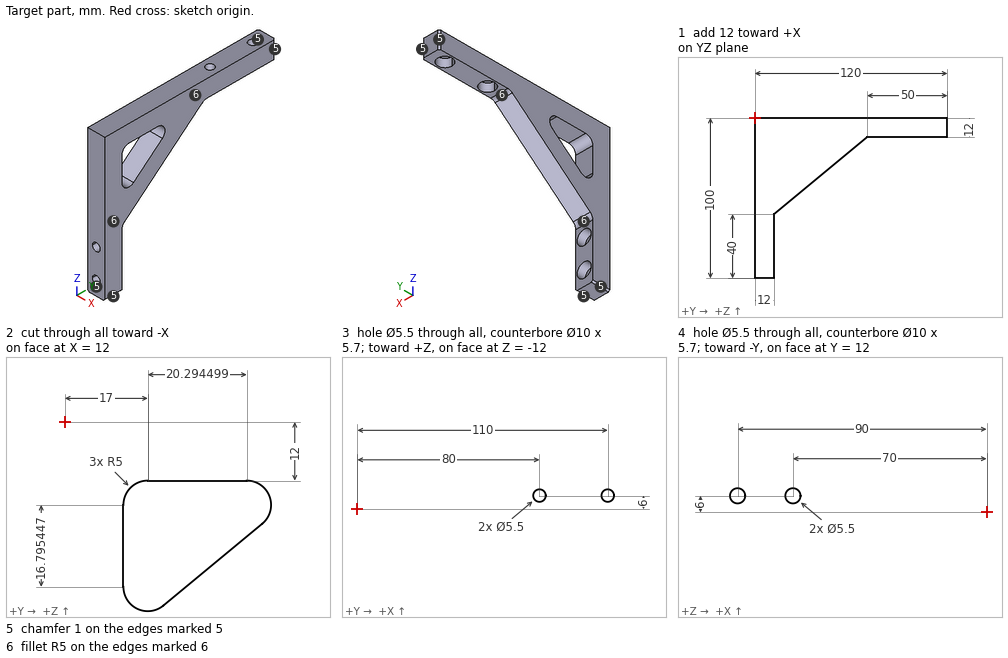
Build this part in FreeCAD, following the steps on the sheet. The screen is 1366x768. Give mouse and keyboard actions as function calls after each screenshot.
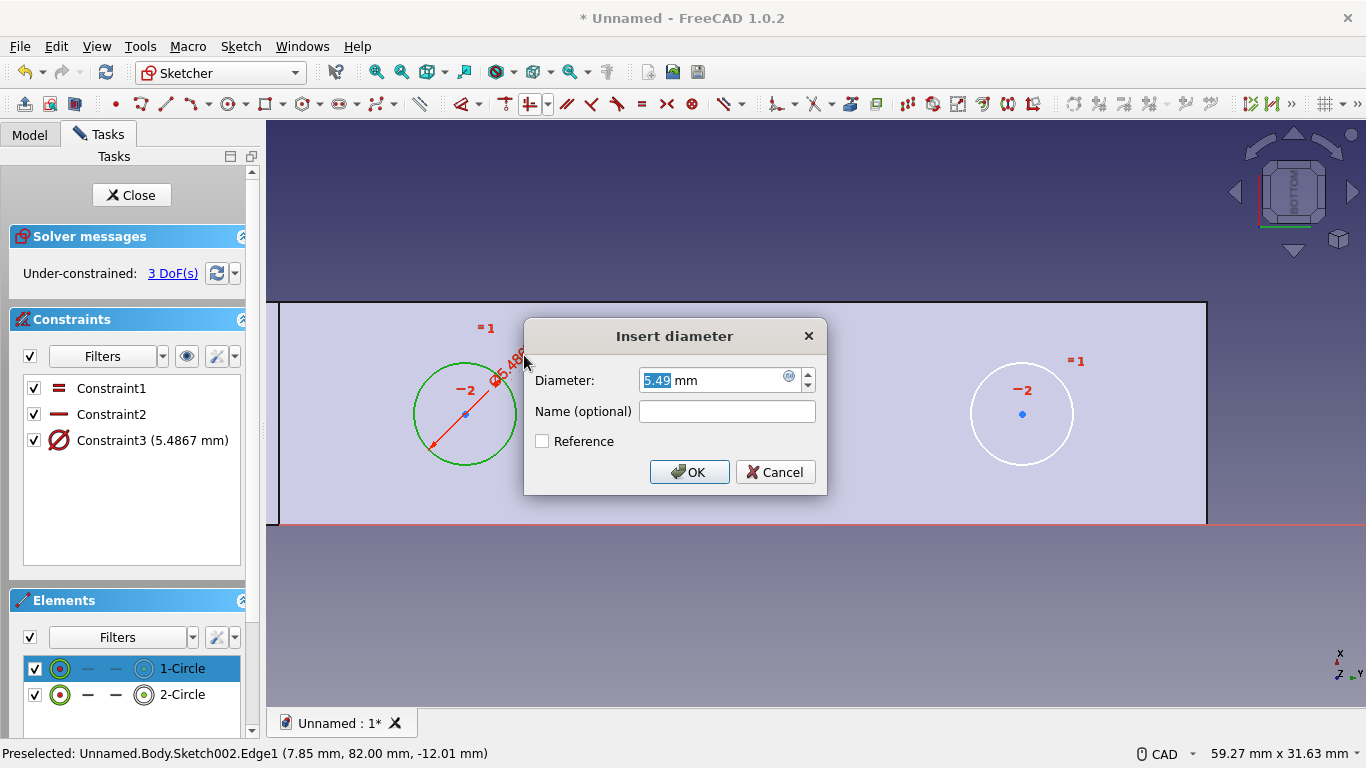
text(5.5)
key(Return)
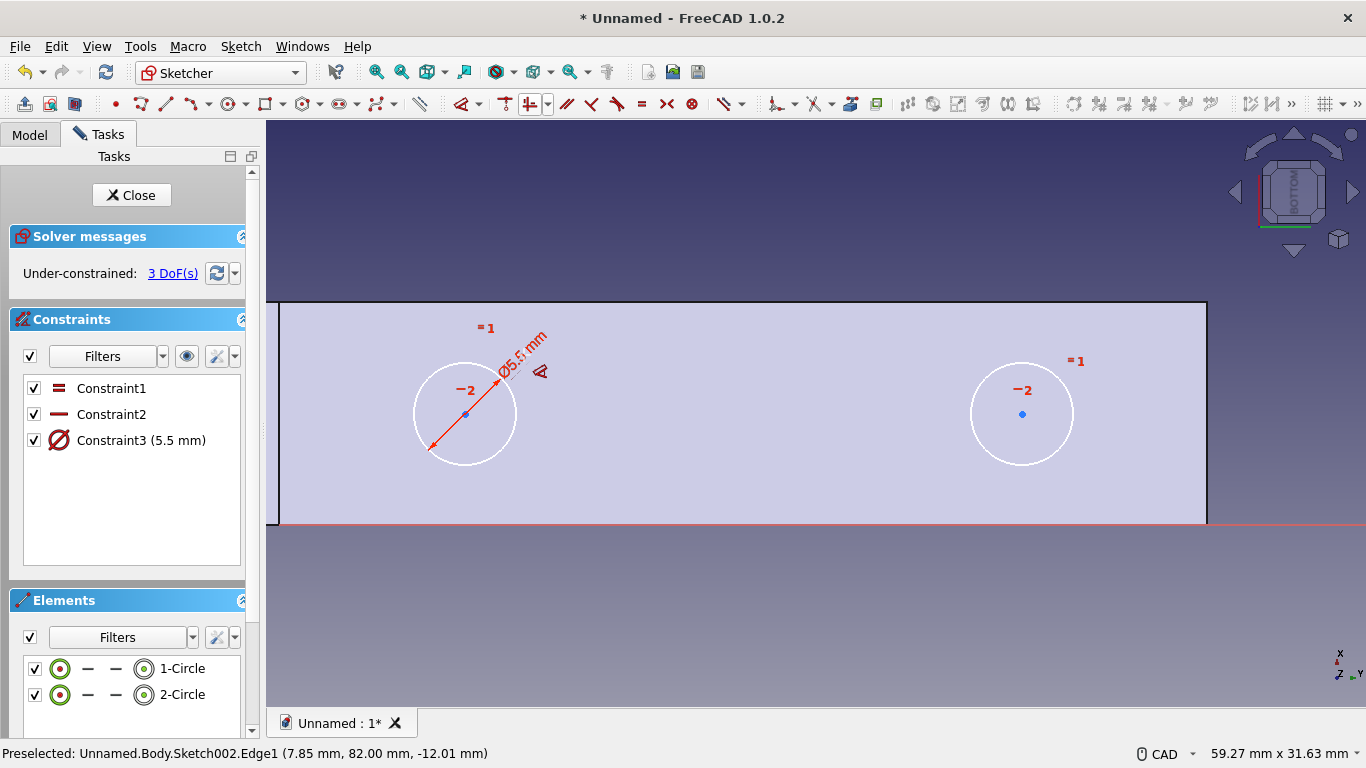
click(465, 414)
click(499, 469)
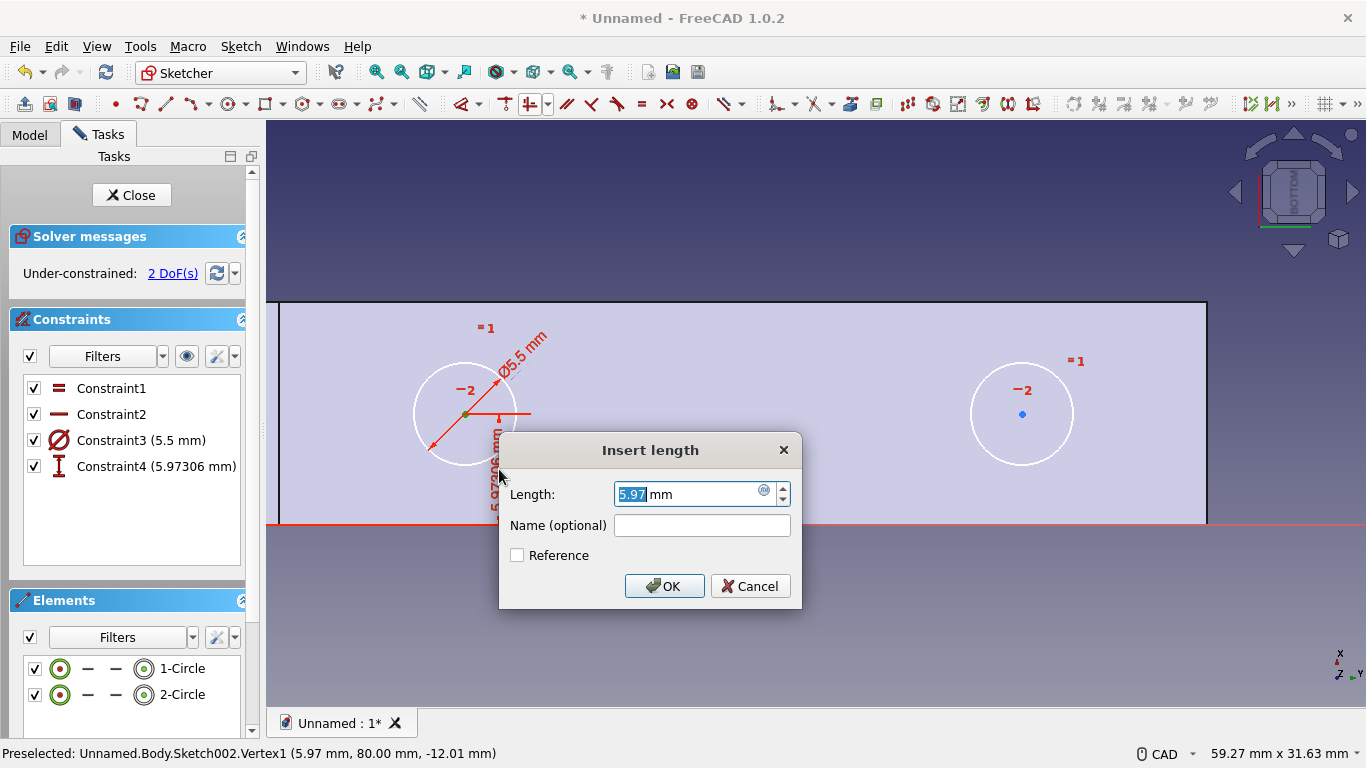
text(6)
key(Return)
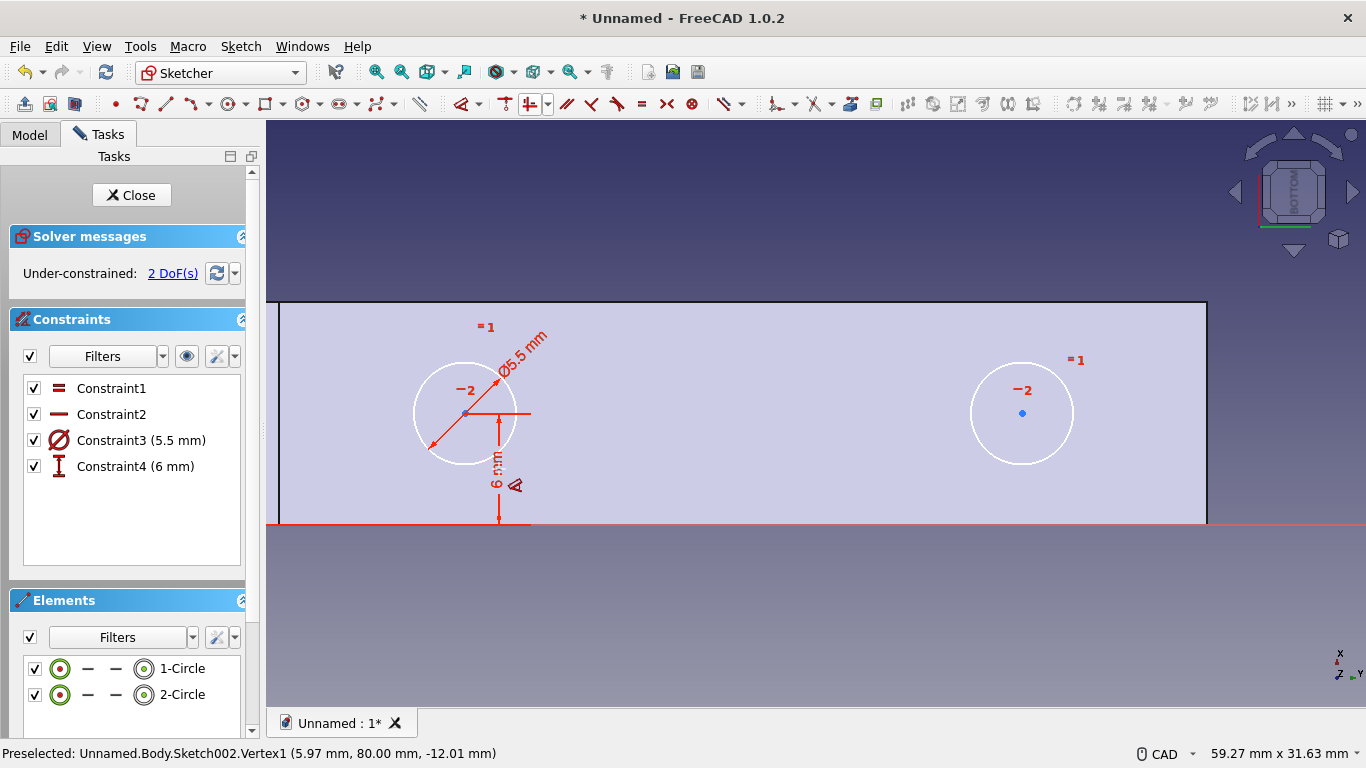
click(465, 413)
click(379, 559)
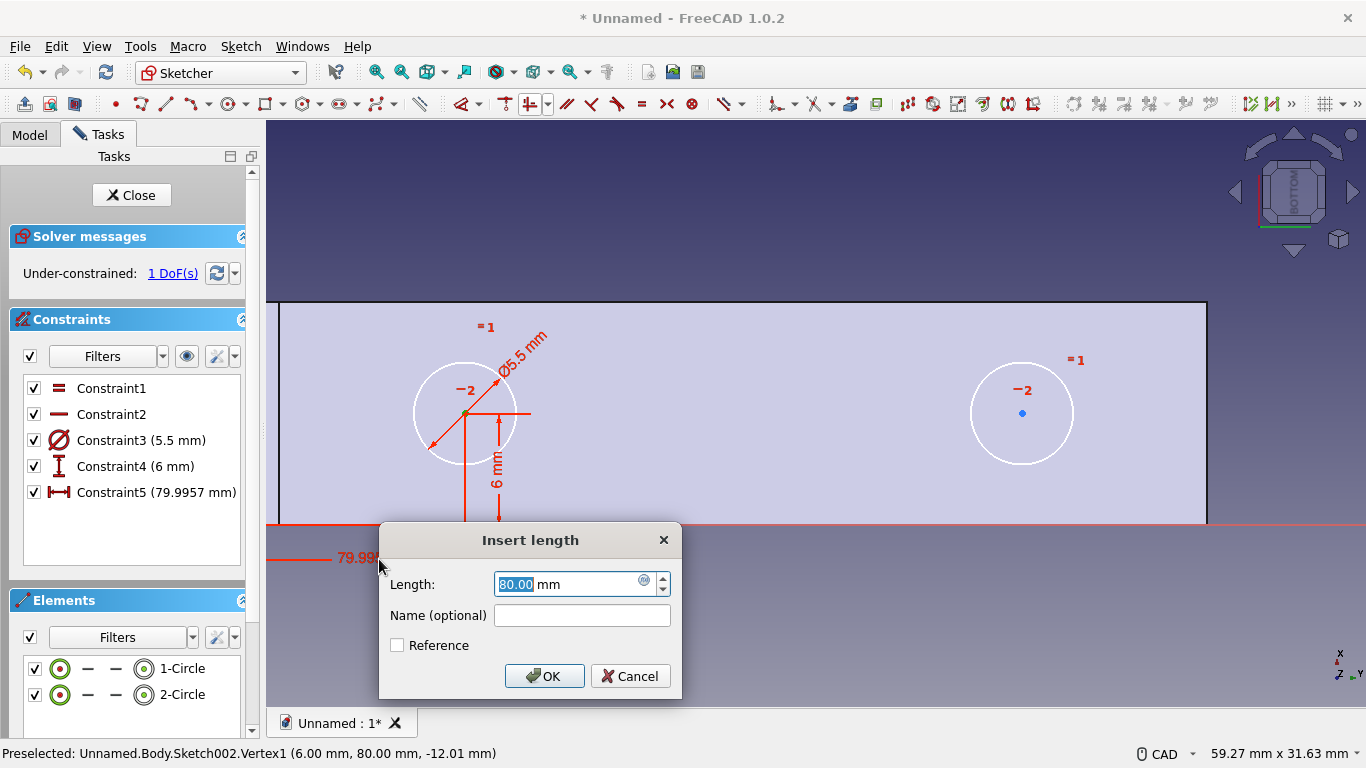
text(80)
key(Return)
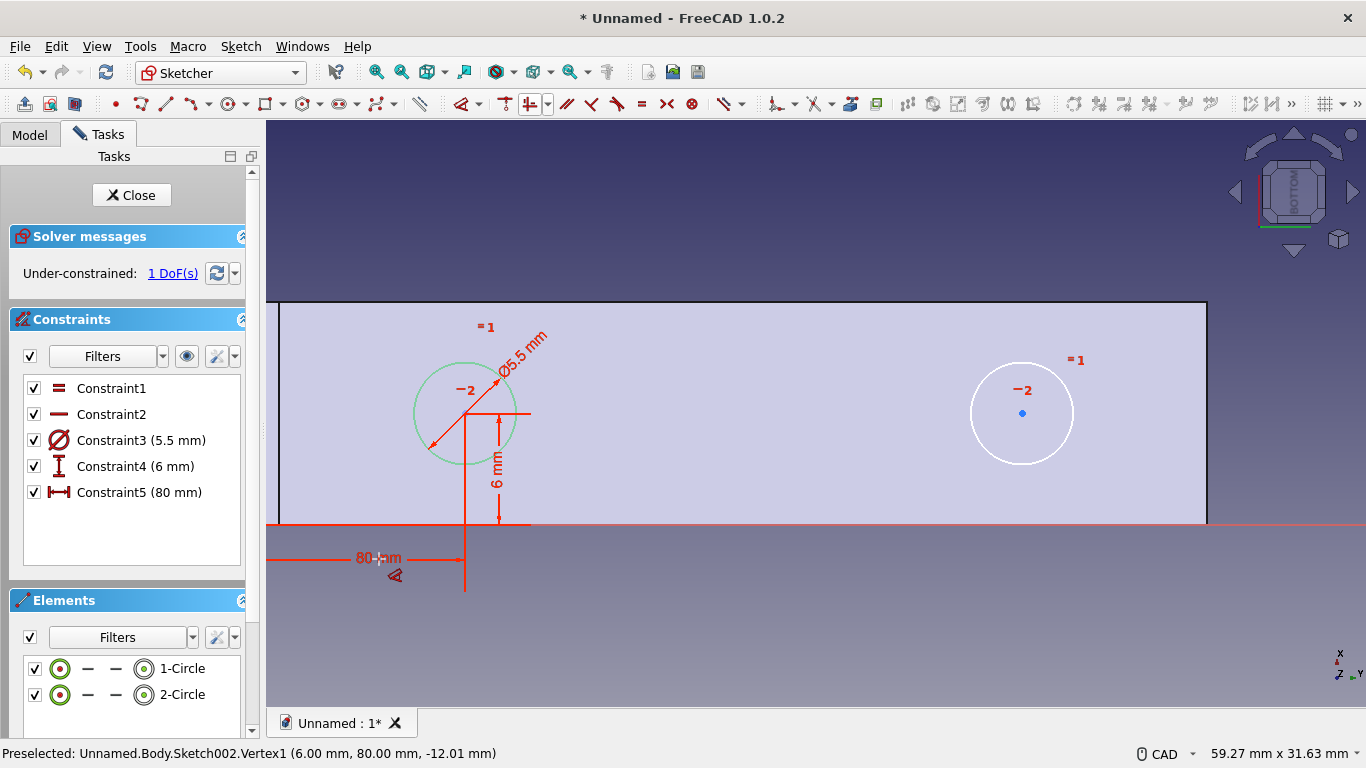
click(1022, 413)
click(658, 559)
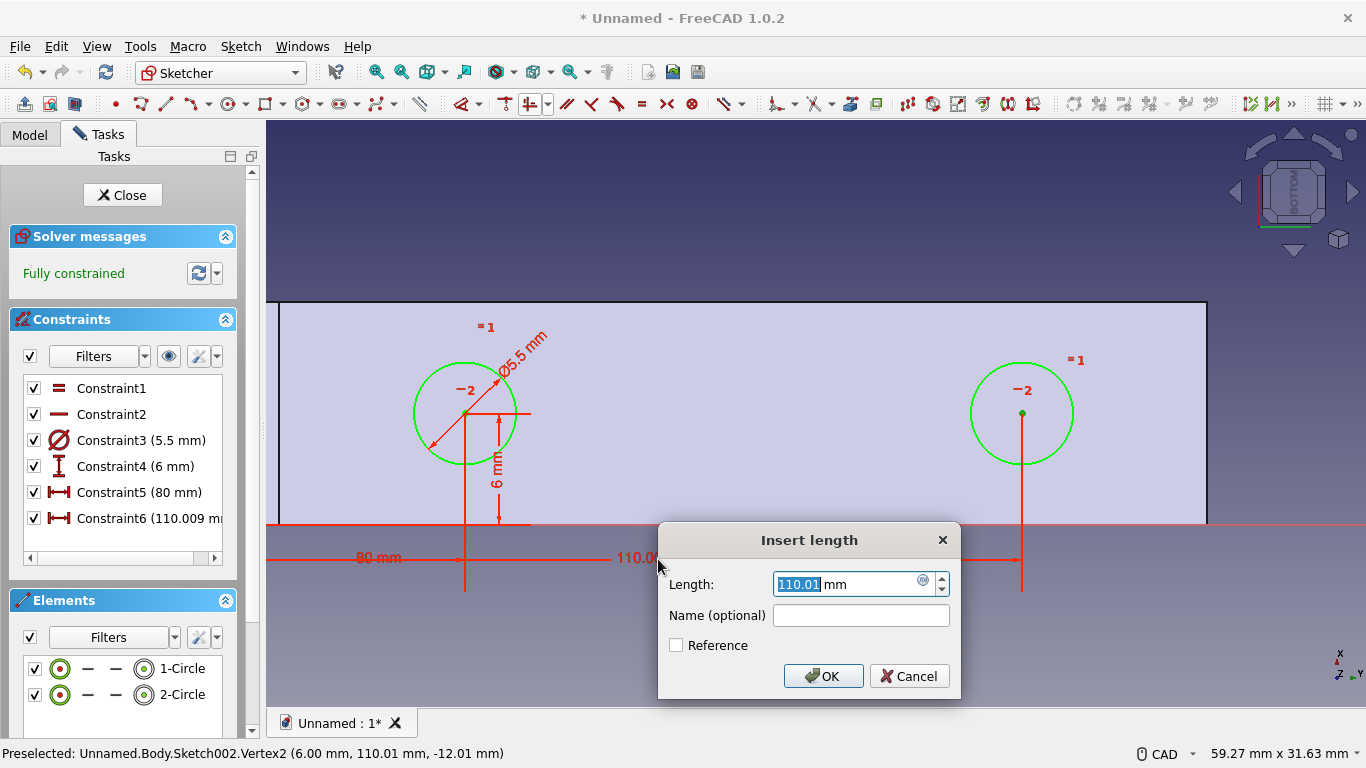
text(110)
key(Return)
key(Escape)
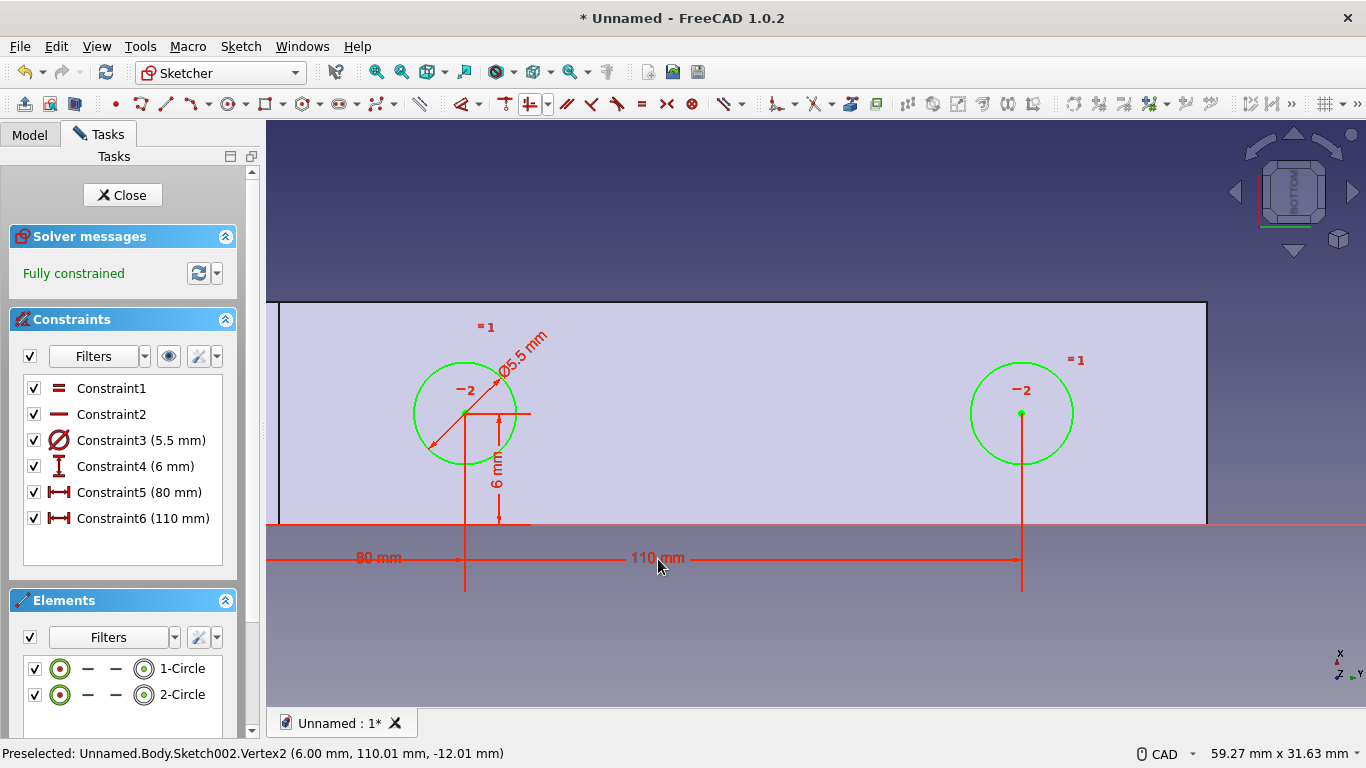
click(123, 195)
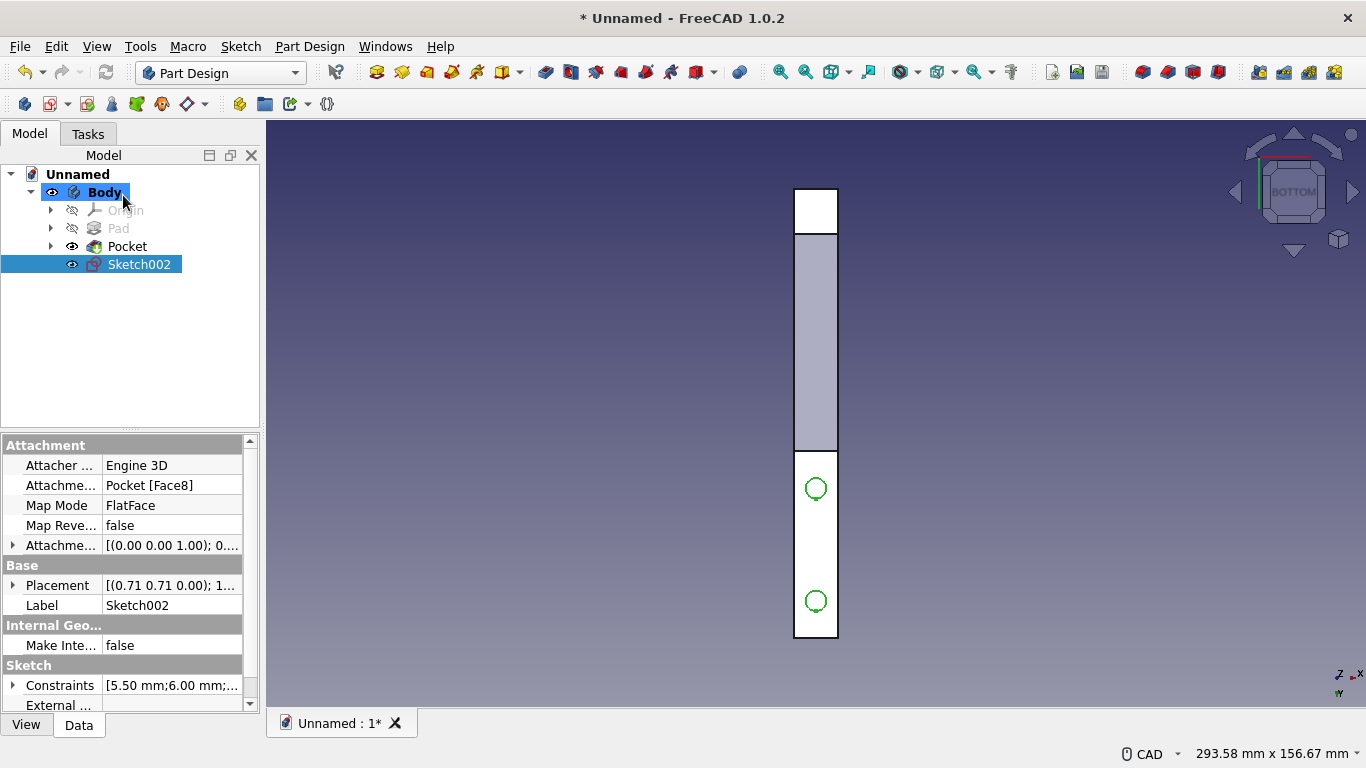
click(571, 72)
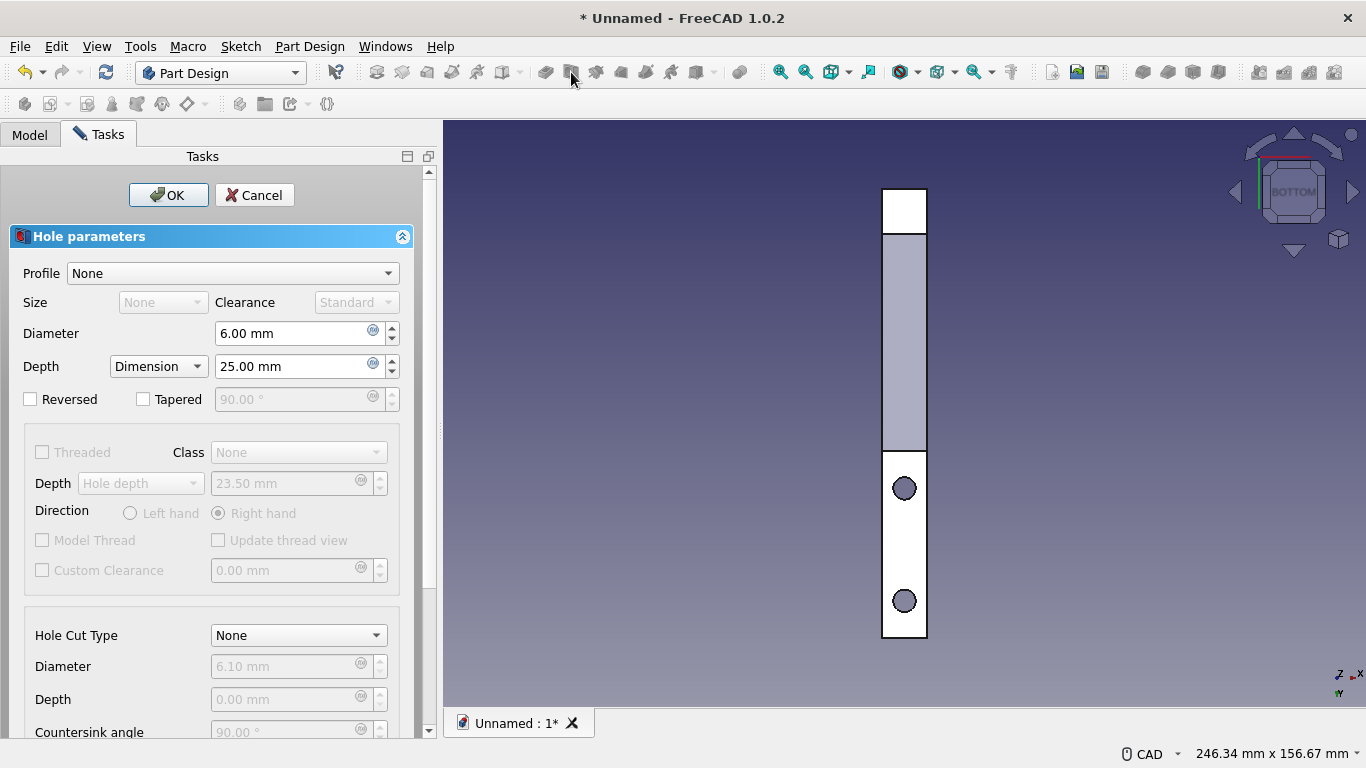
triple_click(300, 334)